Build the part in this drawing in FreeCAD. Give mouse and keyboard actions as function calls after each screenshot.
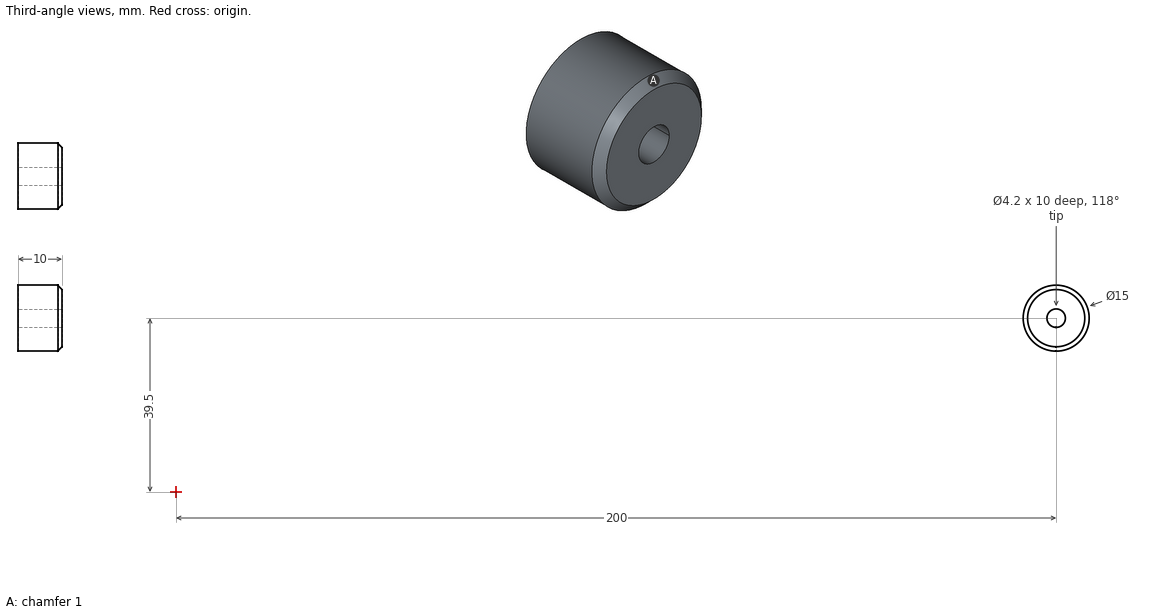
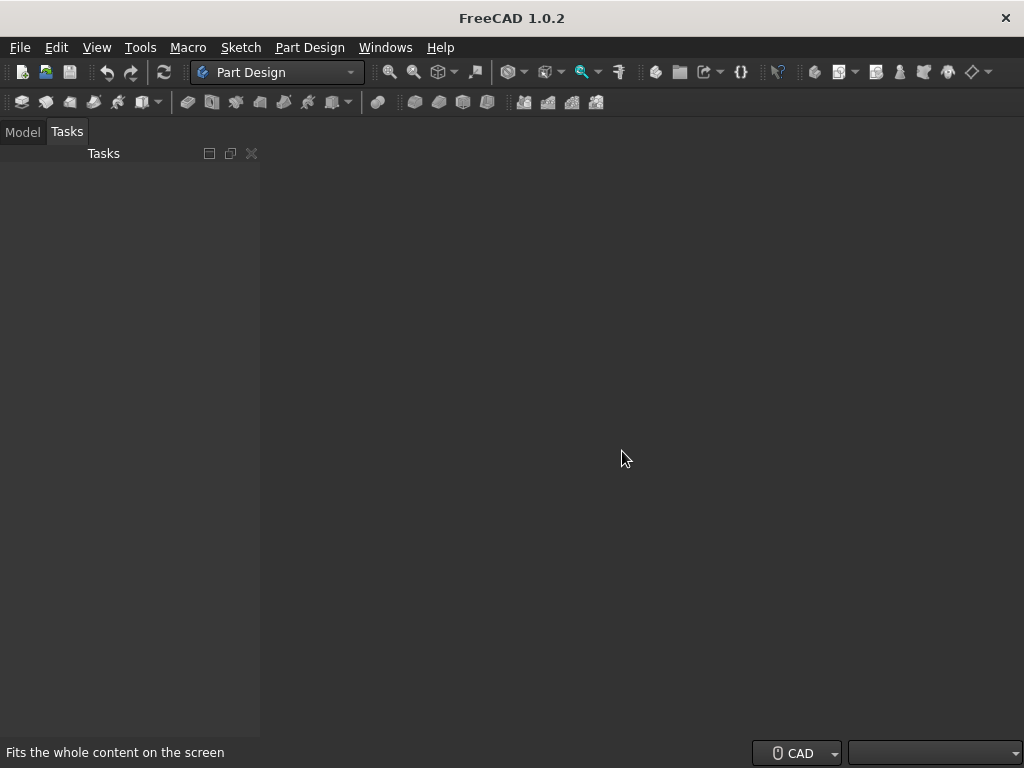
click(22, 72)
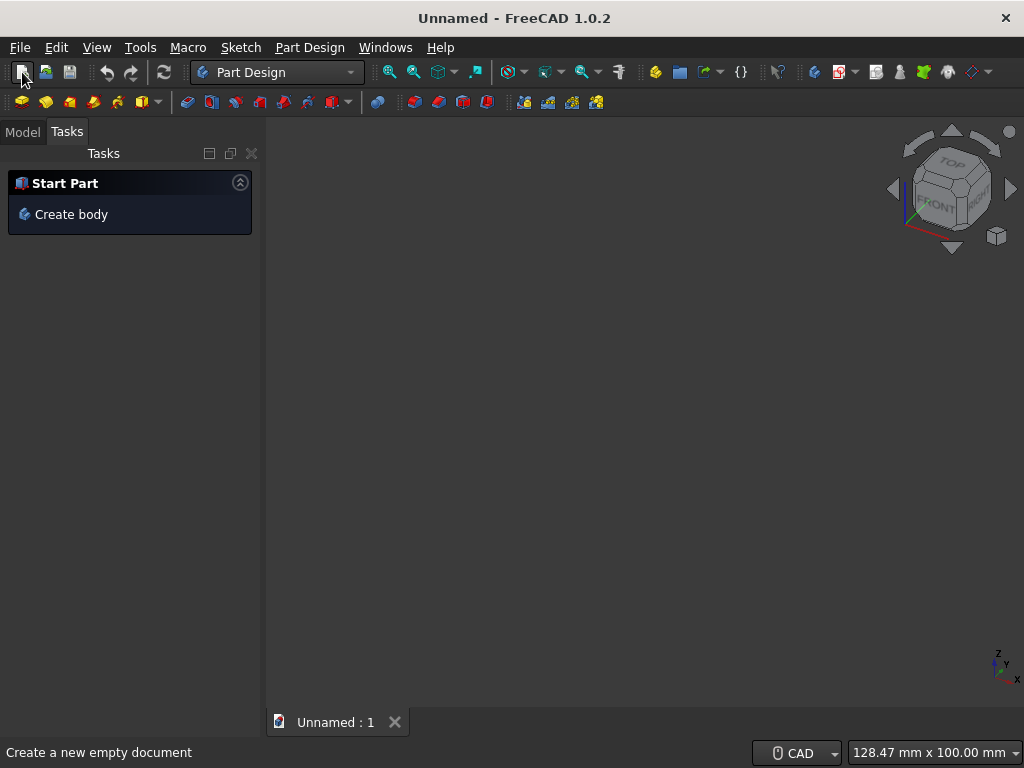
click(816, 72)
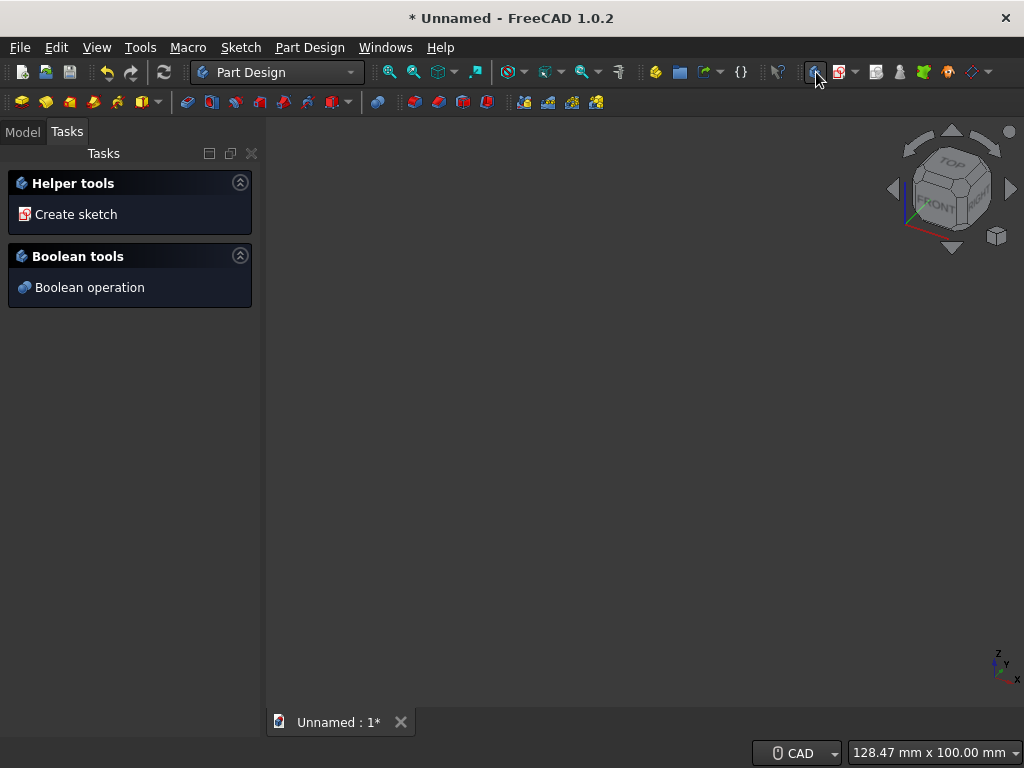
click(23, 131)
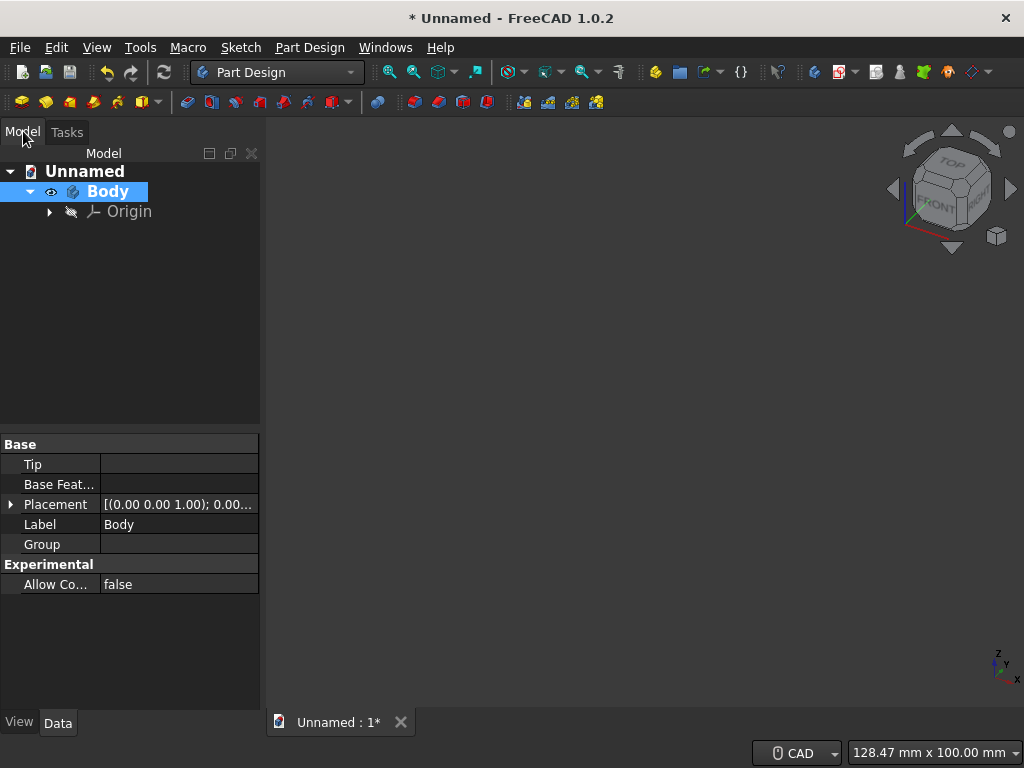
click(50, 212)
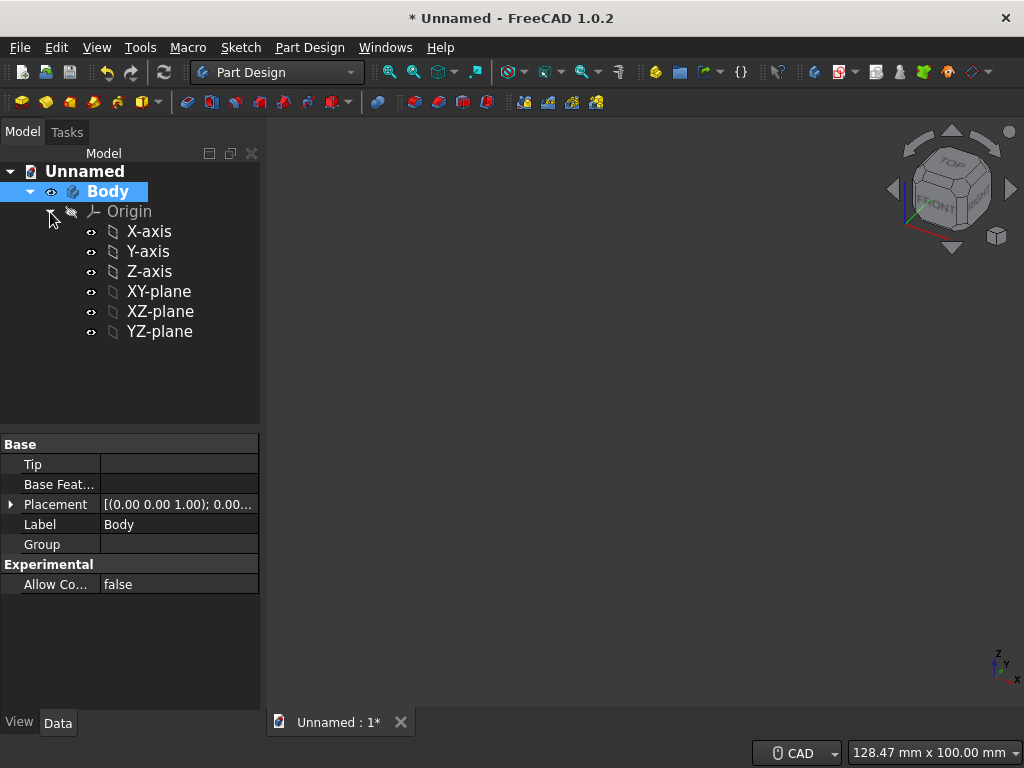
click(136, 332)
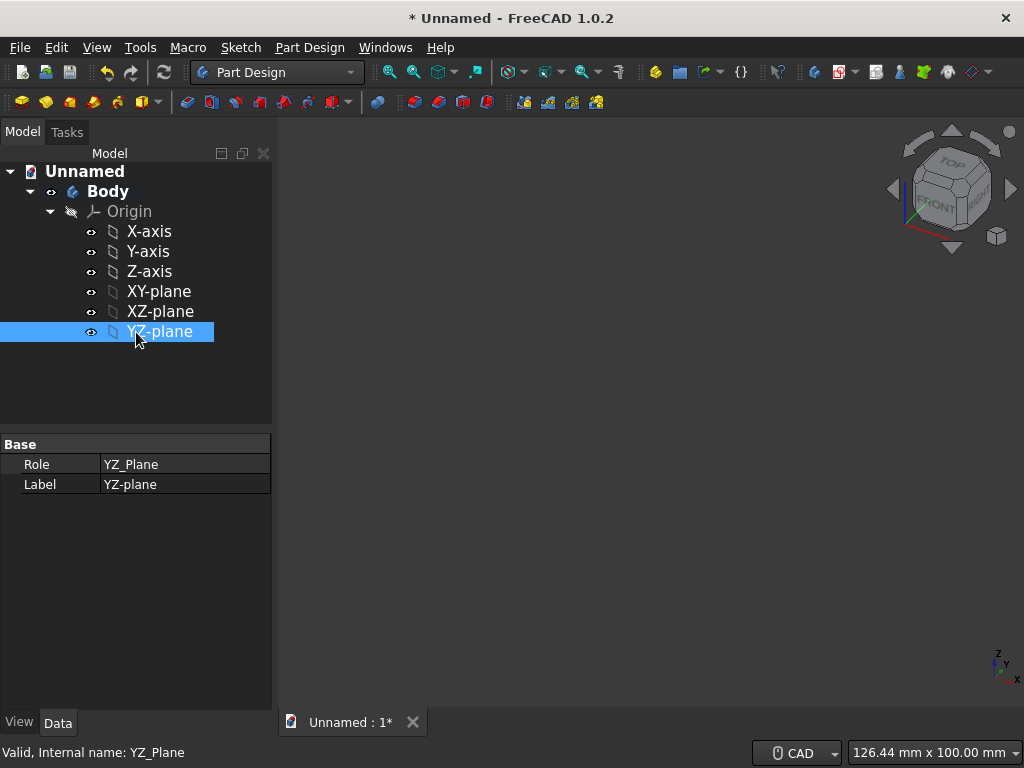
click(972, 72)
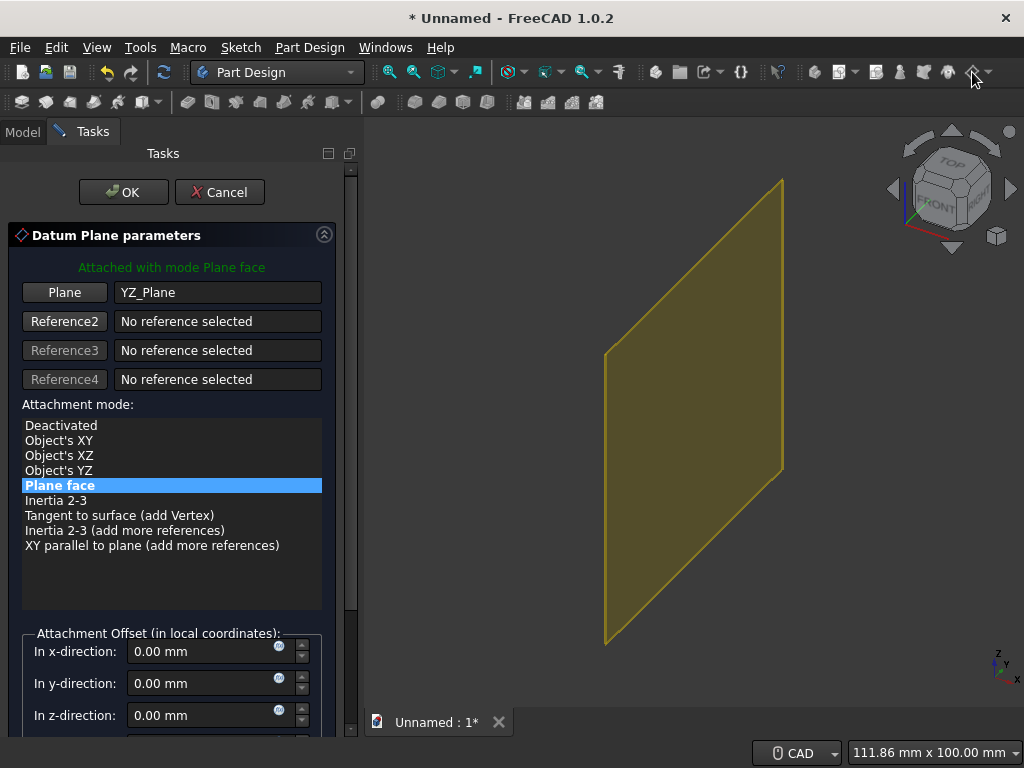
triple_click(210, 715)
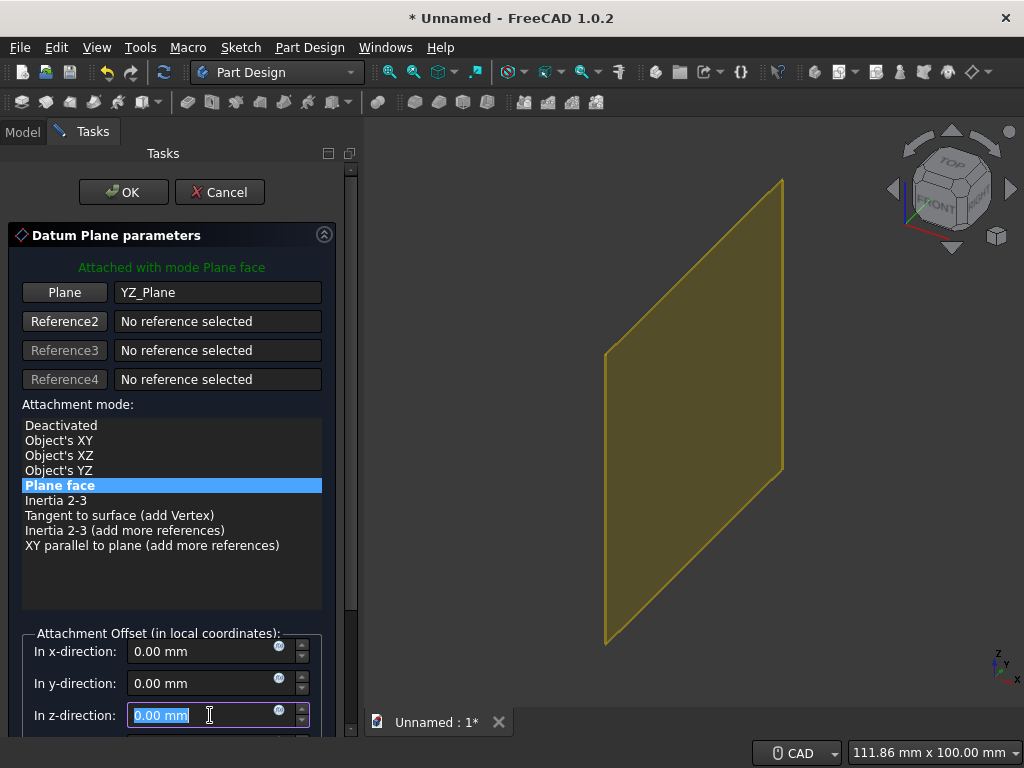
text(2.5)
key(Tab)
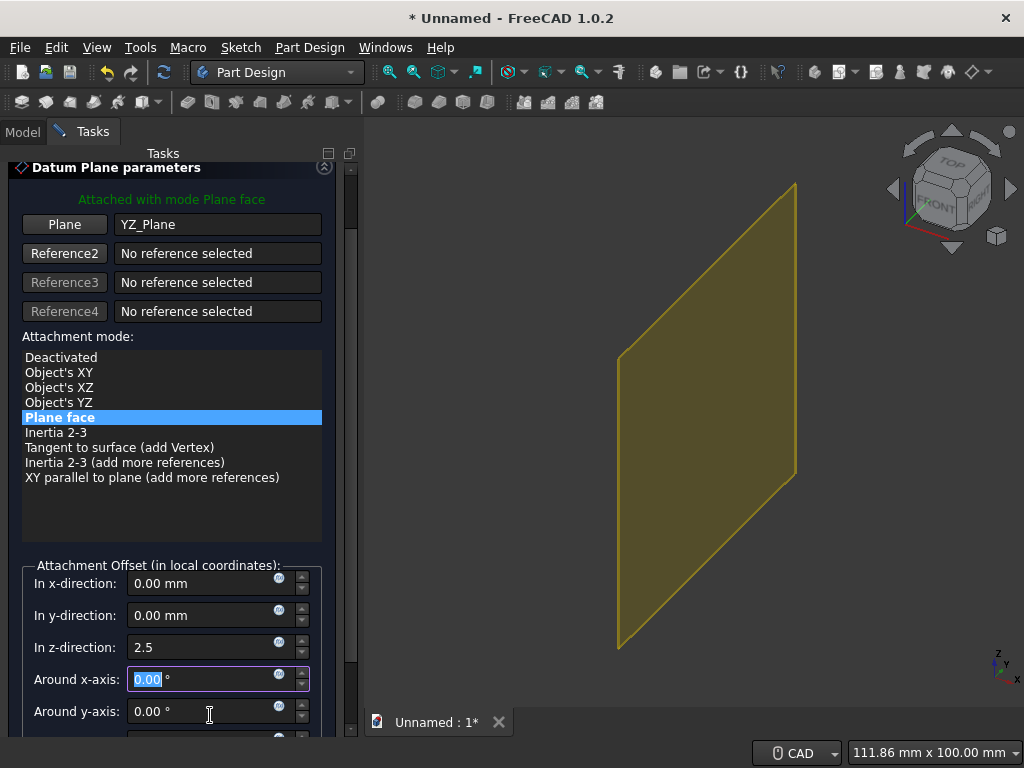
scroll(351, 450, up, 2)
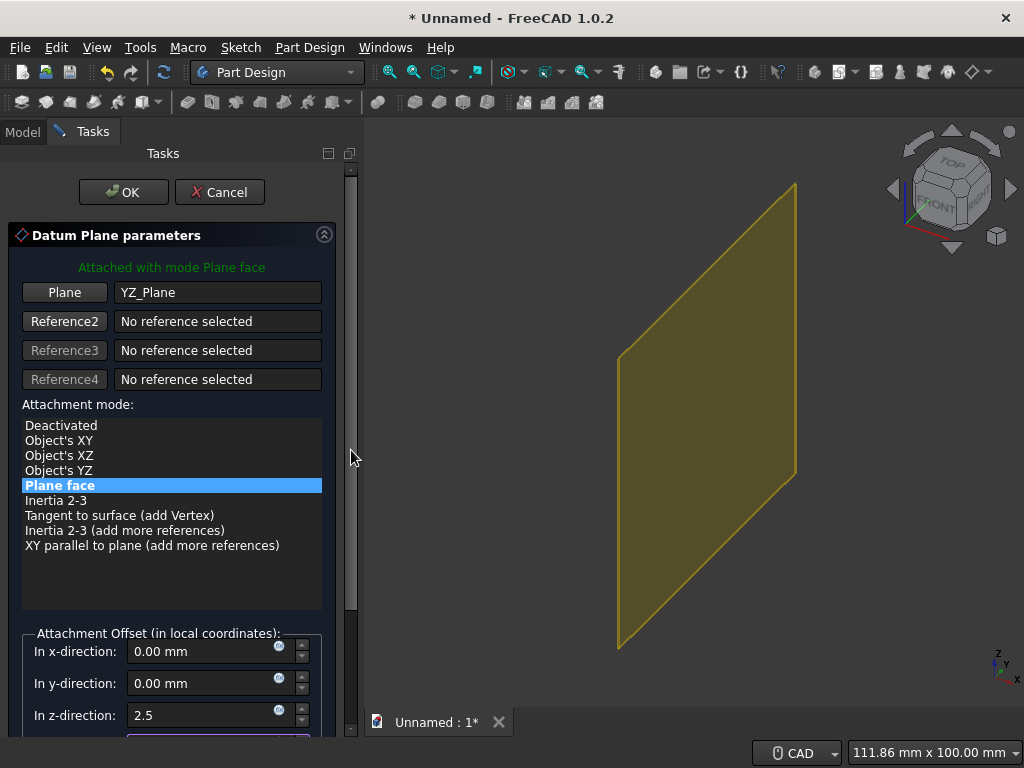
click(124, 192)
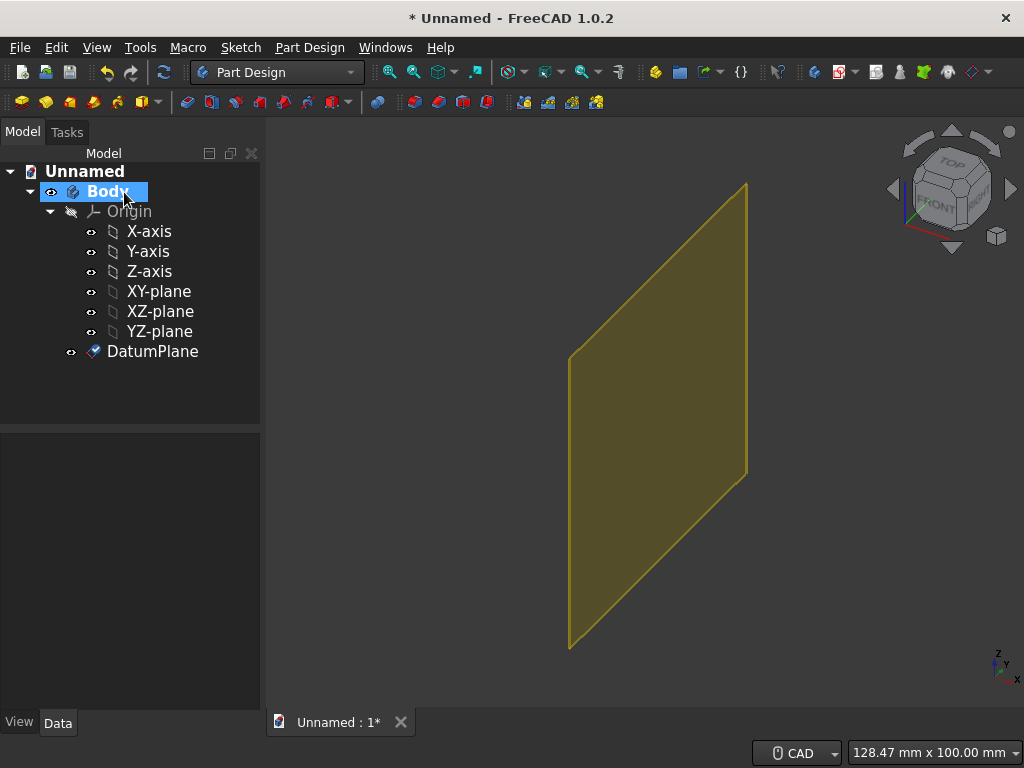
click(116, 352)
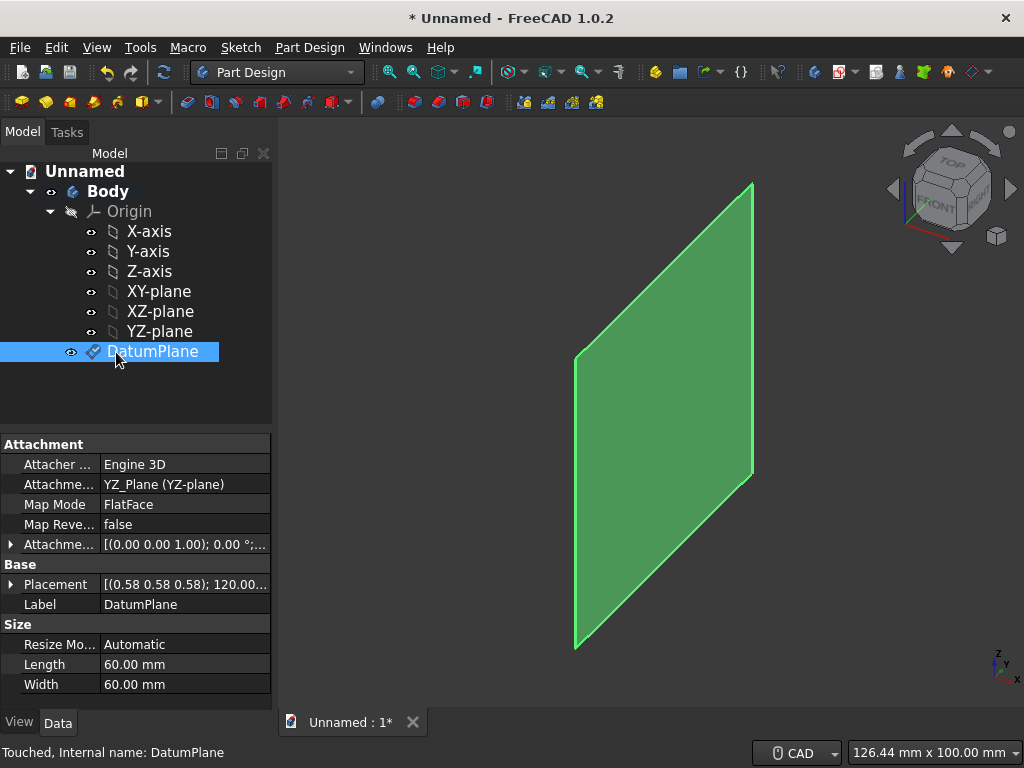
click(840, 72)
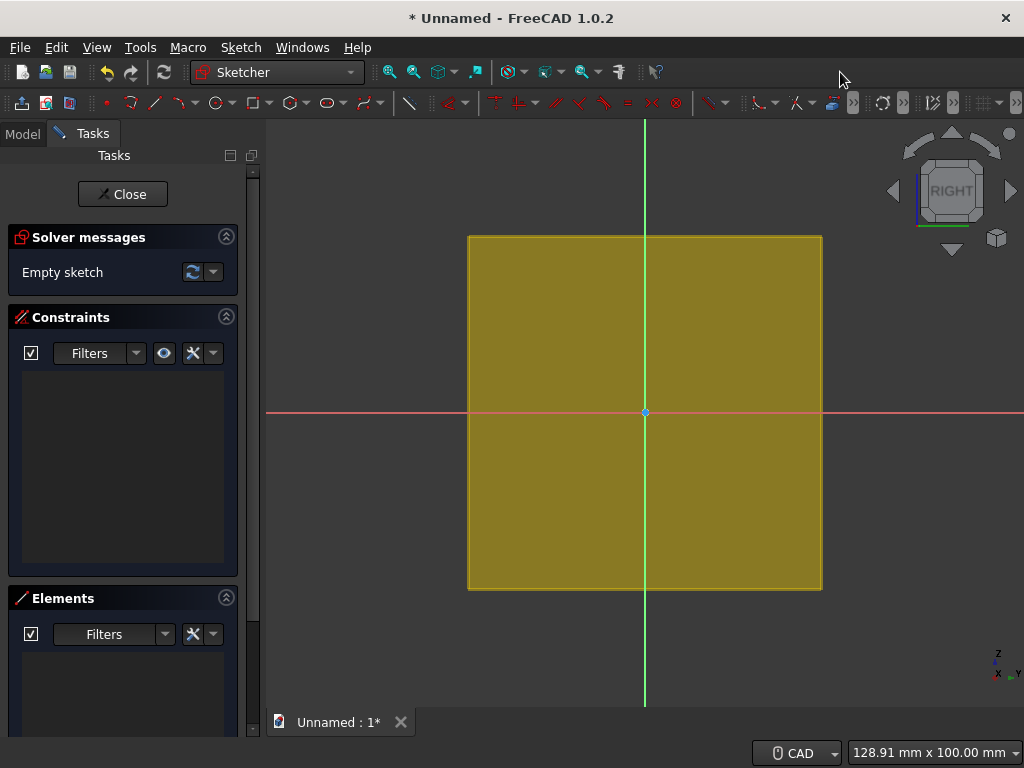
scroll(576, 413, down, 5)